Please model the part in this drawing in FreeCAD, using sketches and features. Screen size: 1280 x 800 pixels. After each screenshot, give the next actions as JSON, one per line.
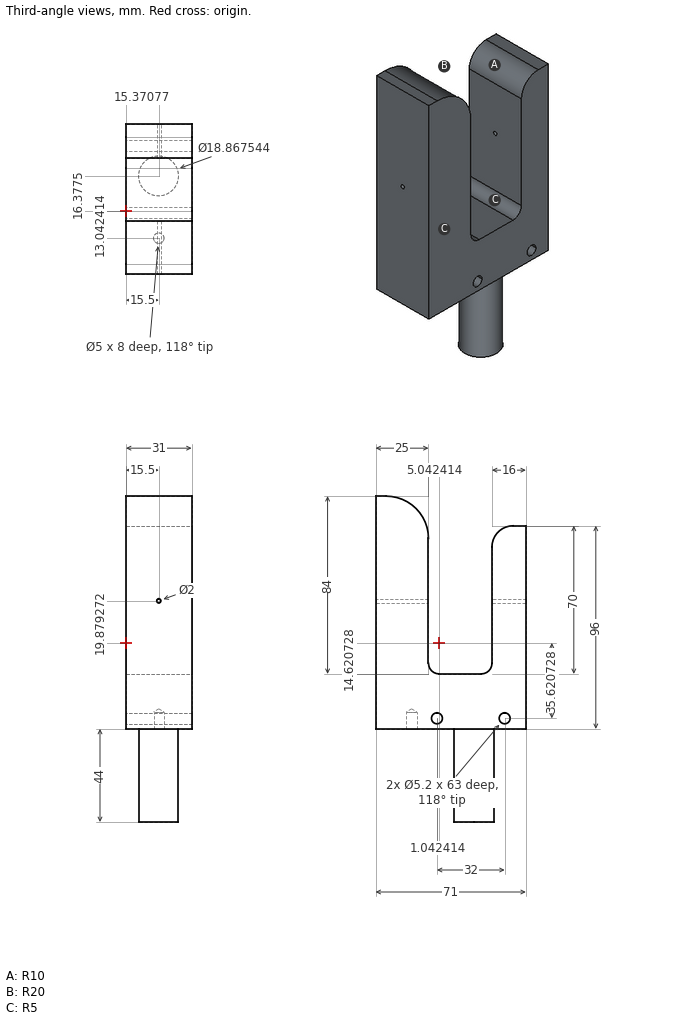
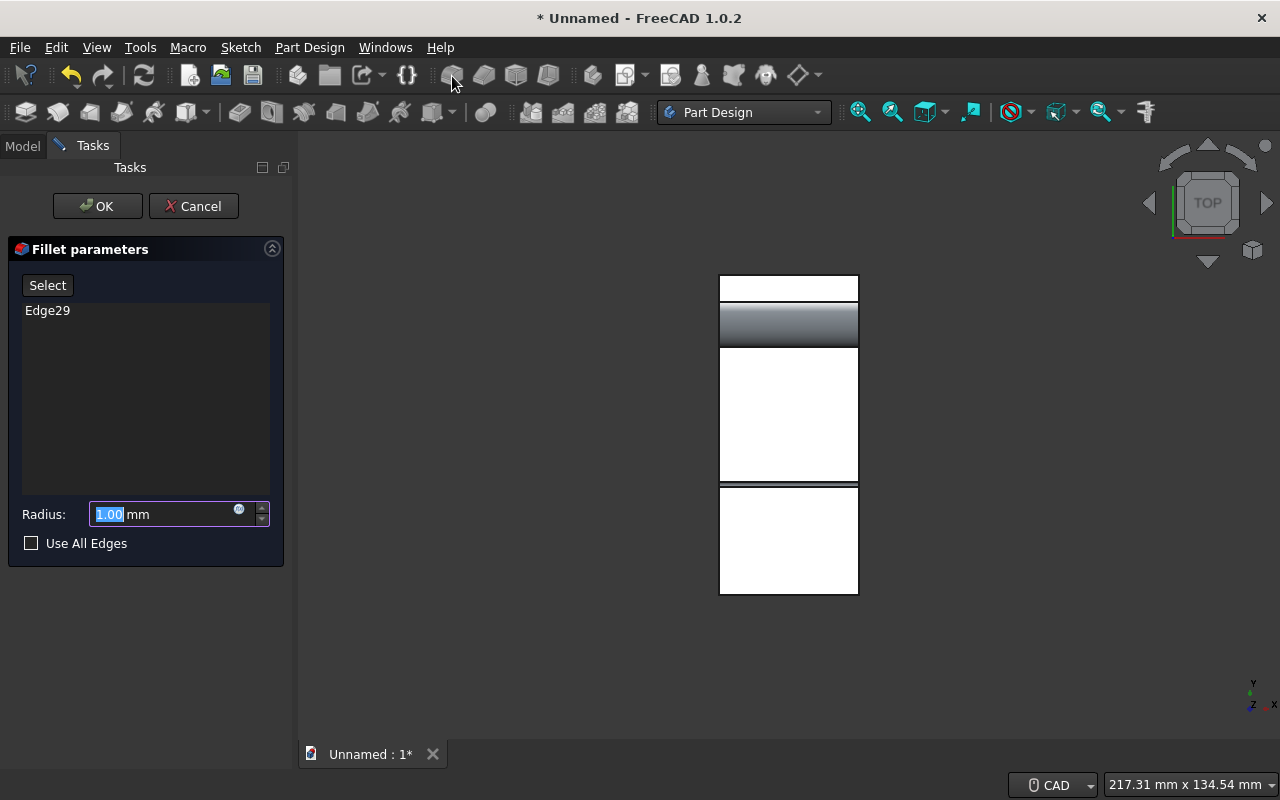
{"action": "type", "text": "20"}
{"action": "key", "text": "Tab"}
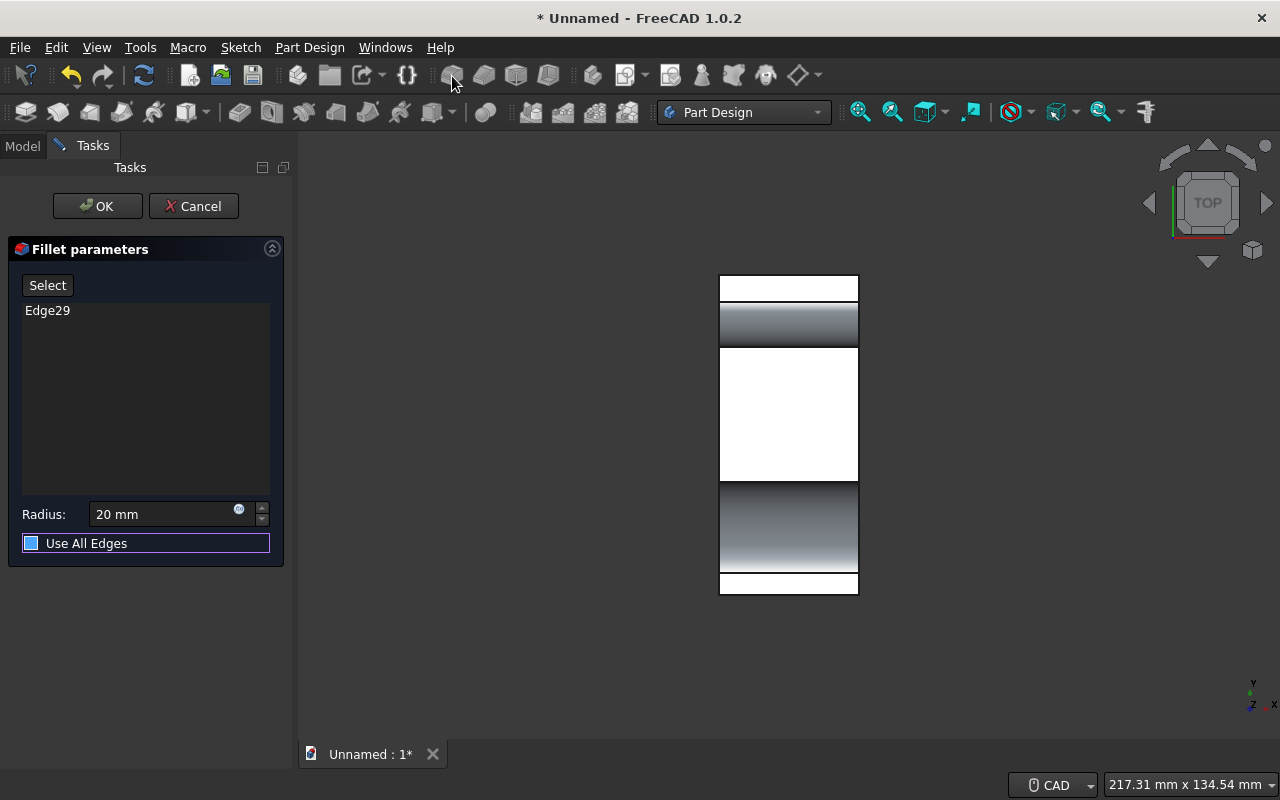
{"action": "left_click", "coordinate": [98, 206]}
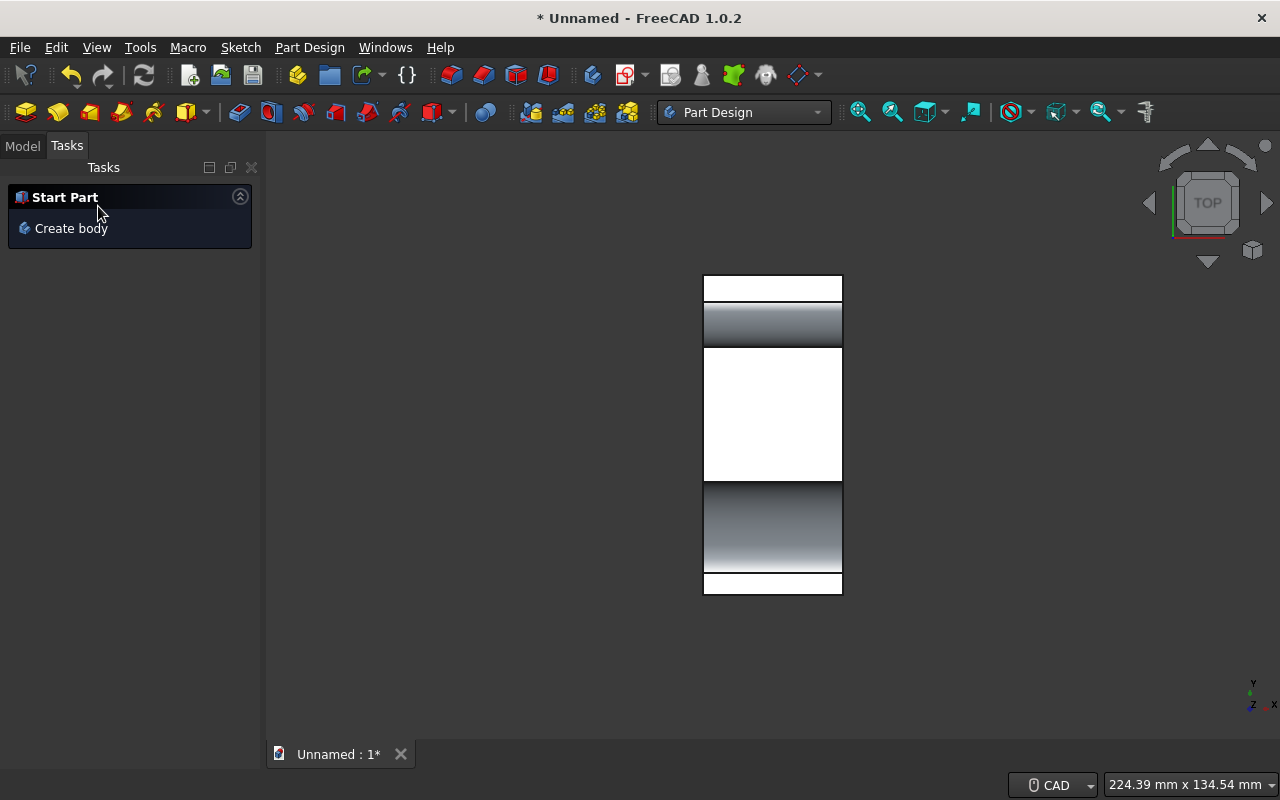
{"action": "key", "text": "0"}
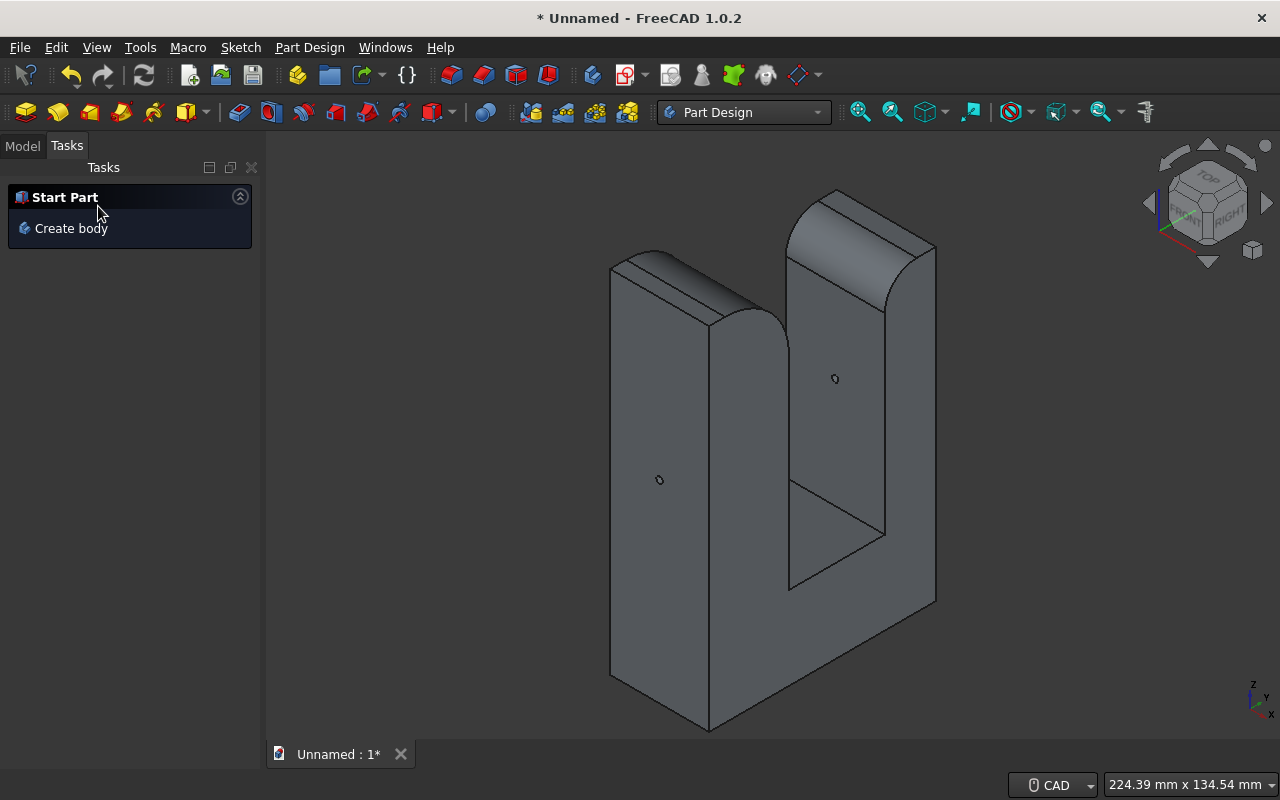
{"action": "key", "text": "2"}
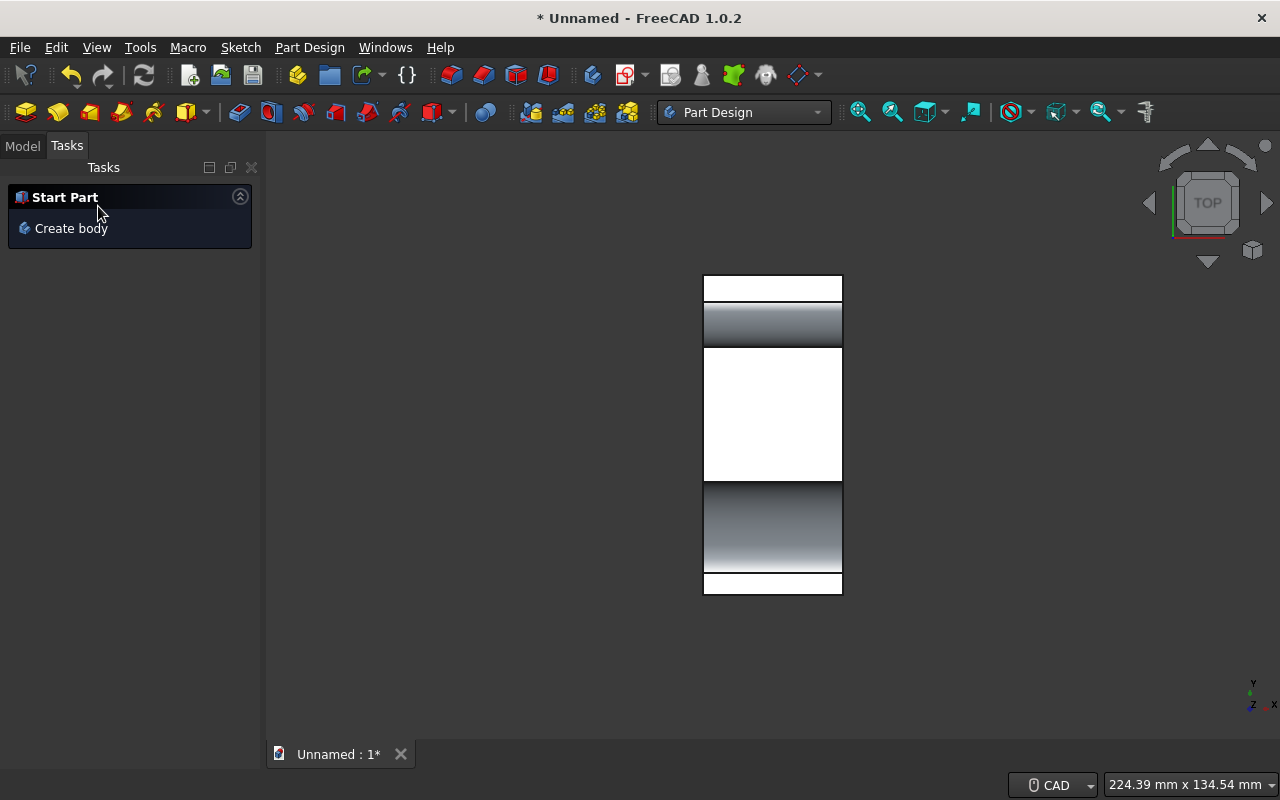
{"action": "key", "text": "1"}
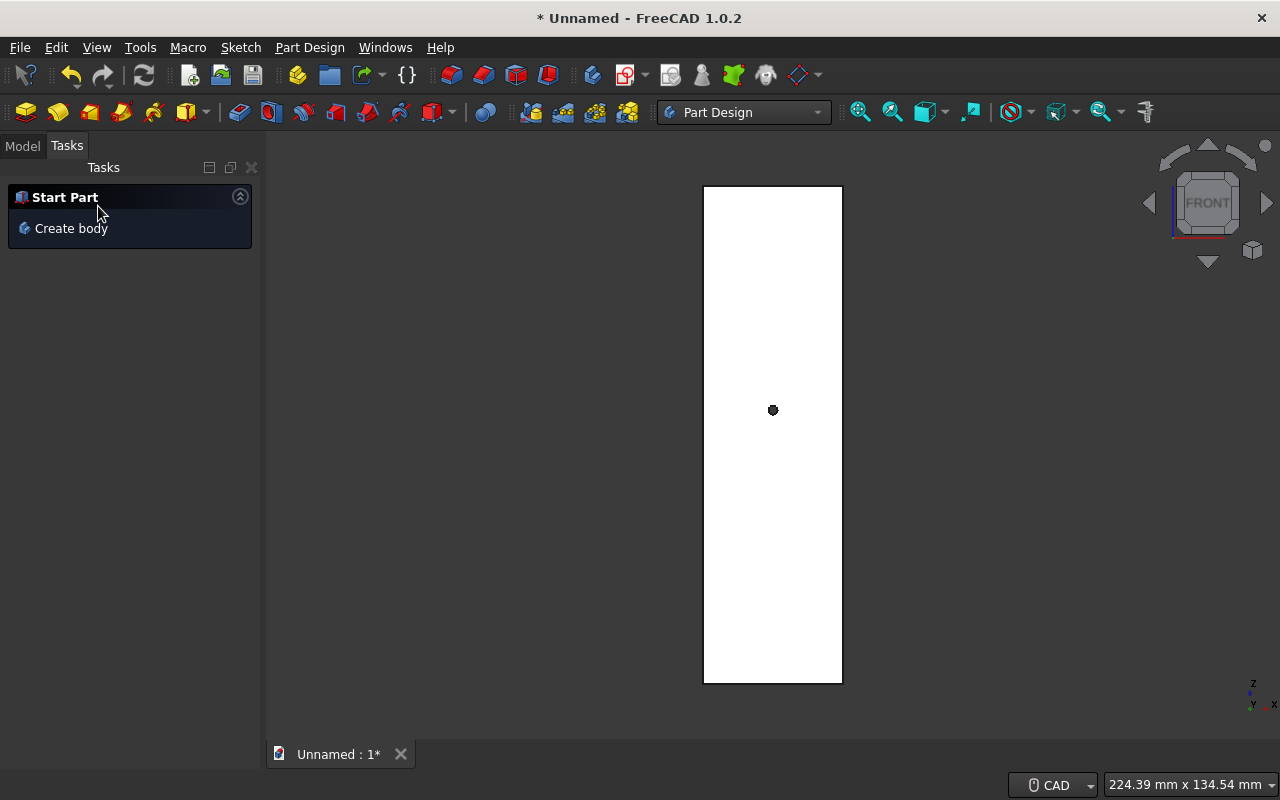
{"action": "key", "text": "3"}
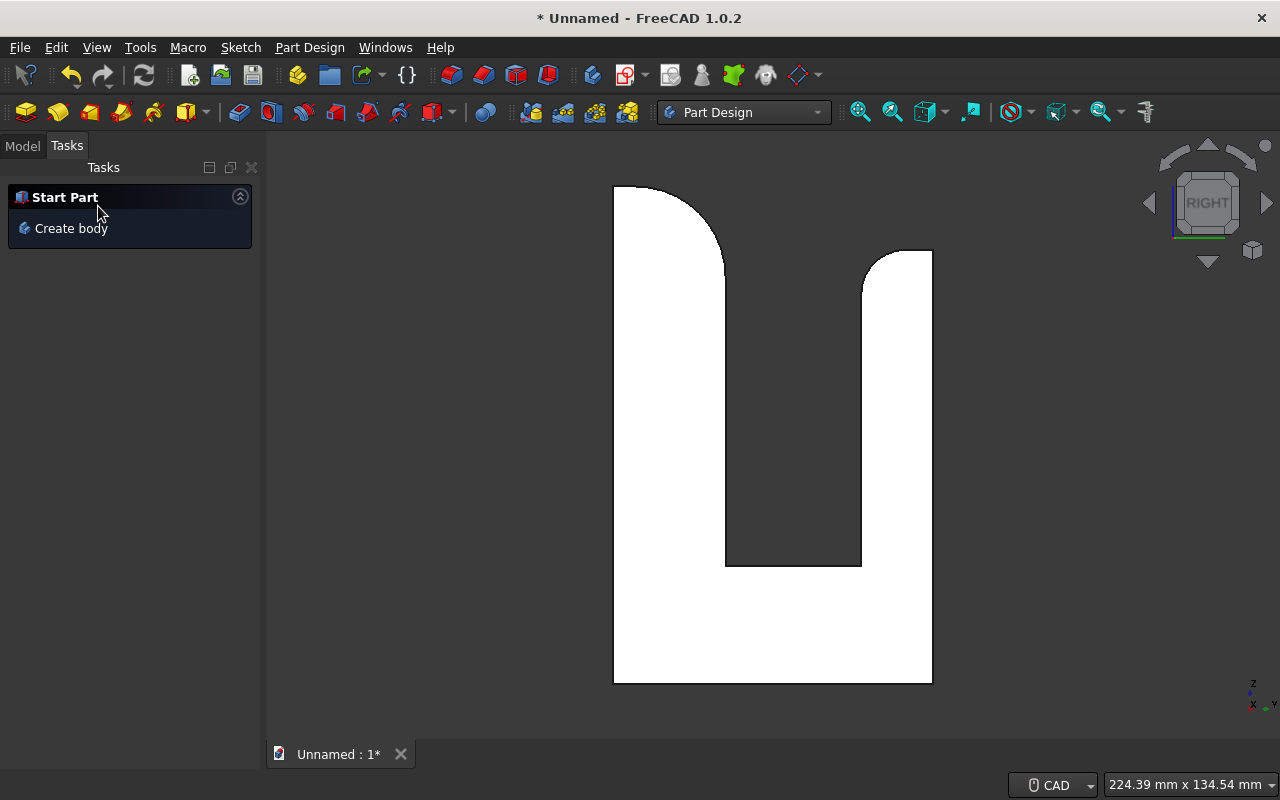
{"action": "key", "text": "5"}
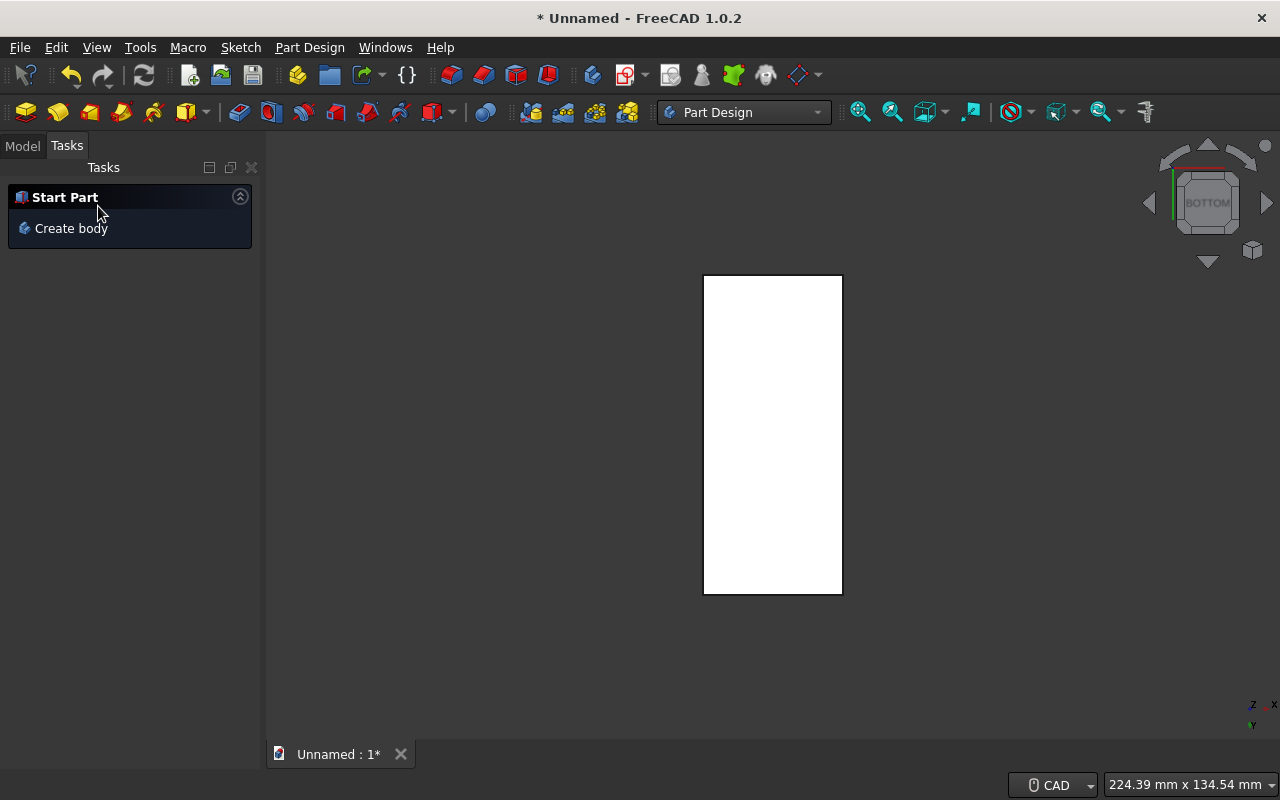
{"action": "key", "text": "4"}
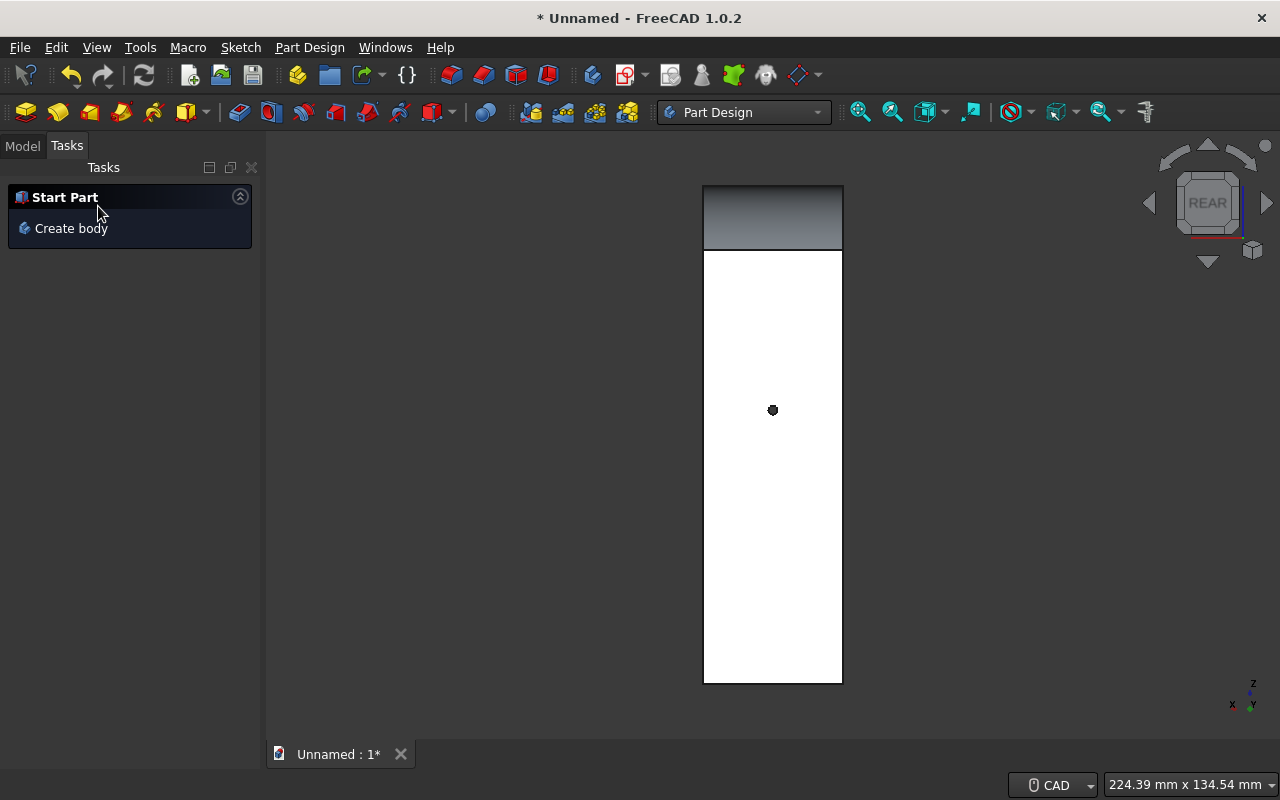
{"action": "key", "text": "6"}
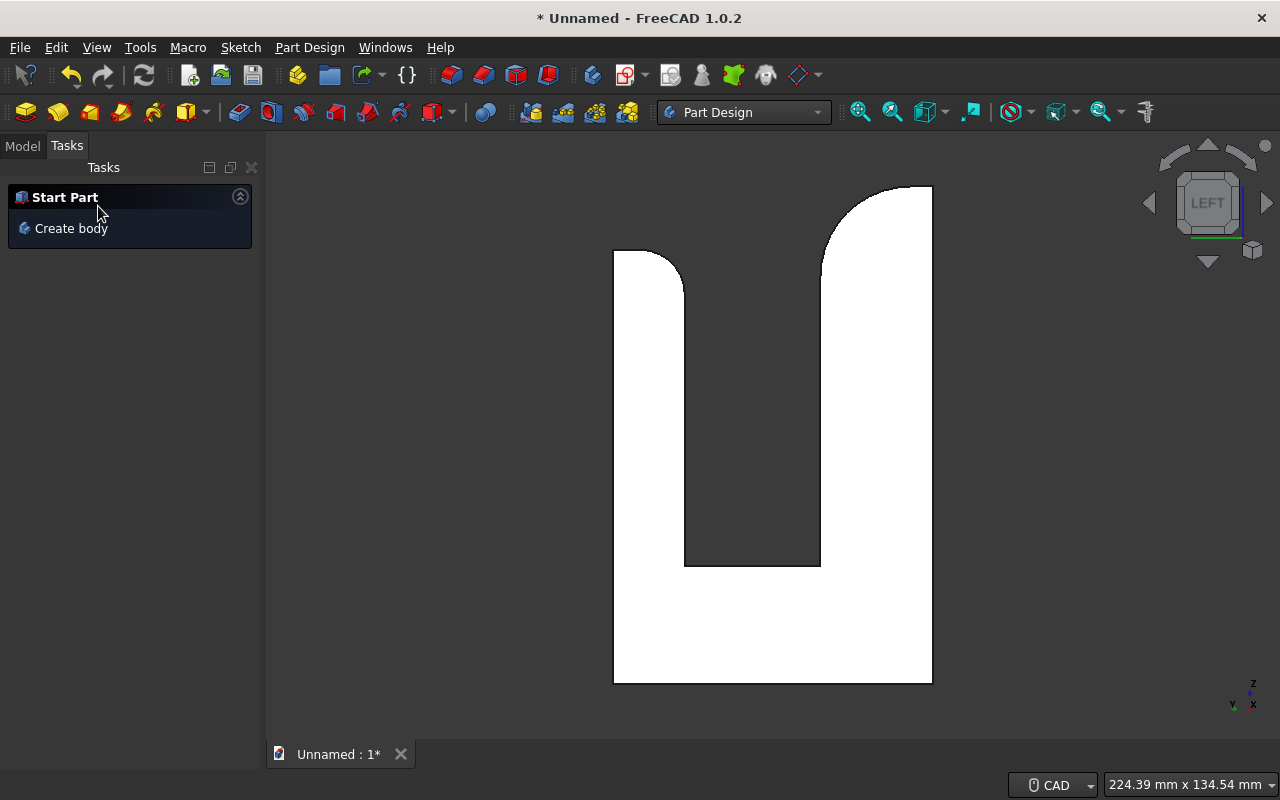
{"action": "key", "text": "v 3"}